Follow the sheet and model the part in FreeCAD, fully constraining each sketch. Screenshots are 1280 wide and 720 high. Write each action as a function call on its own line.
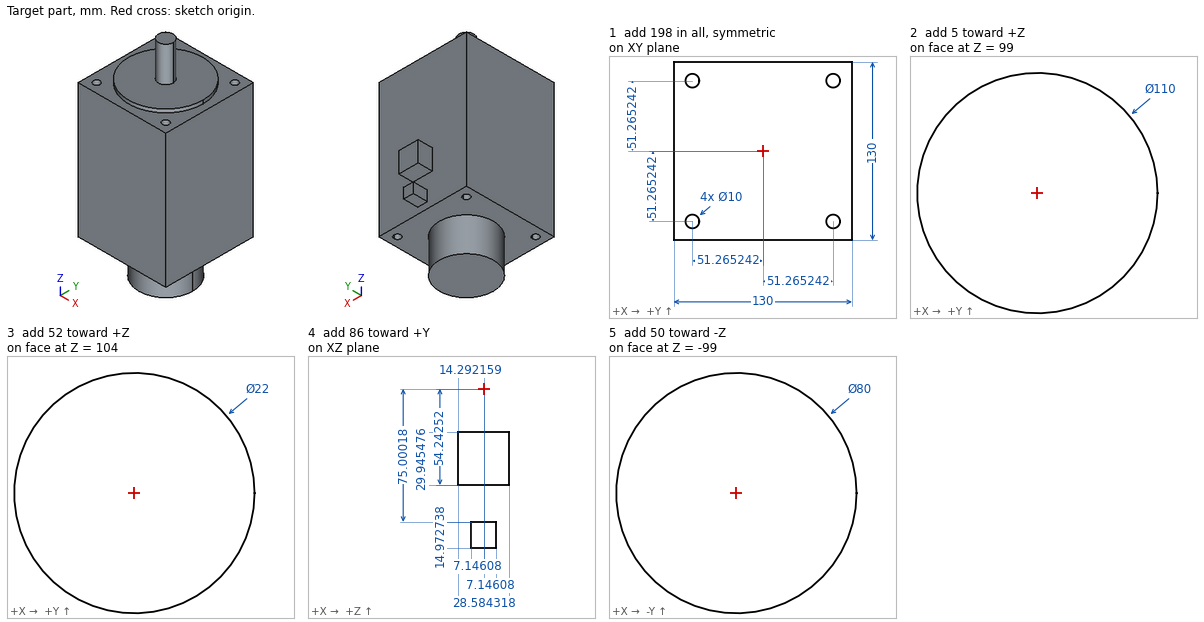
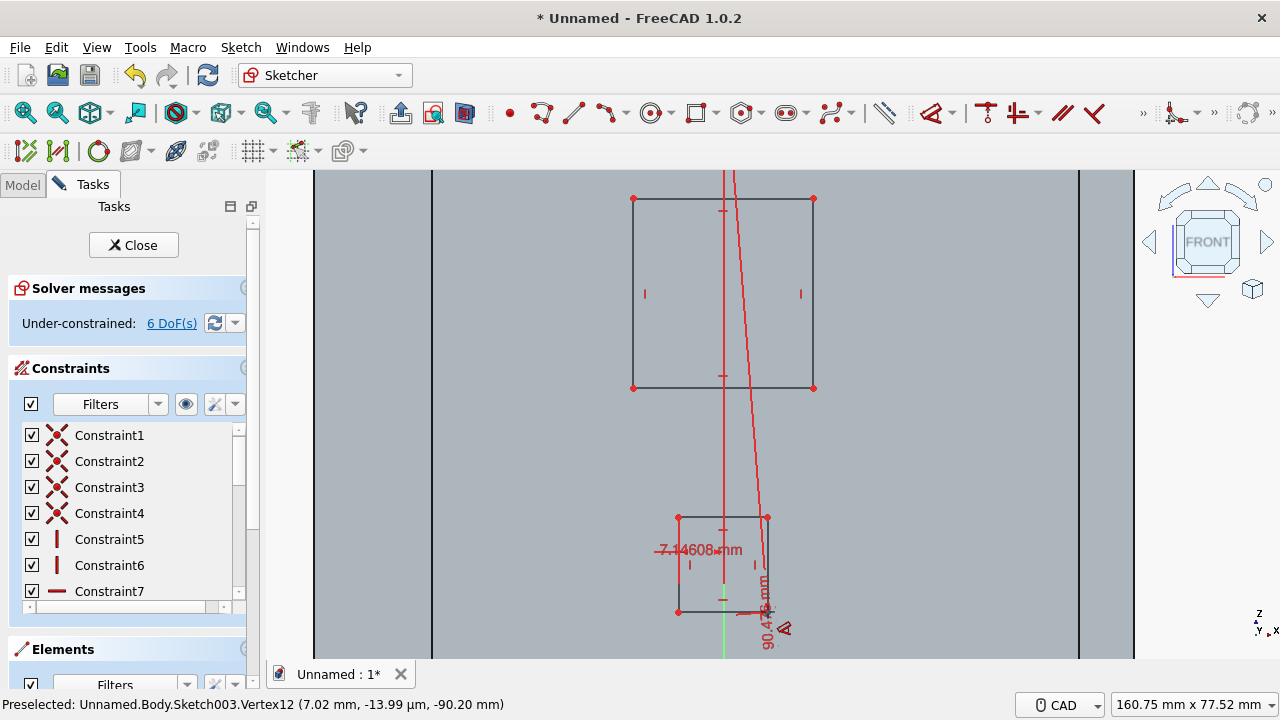
key(Escape)
key(Escape)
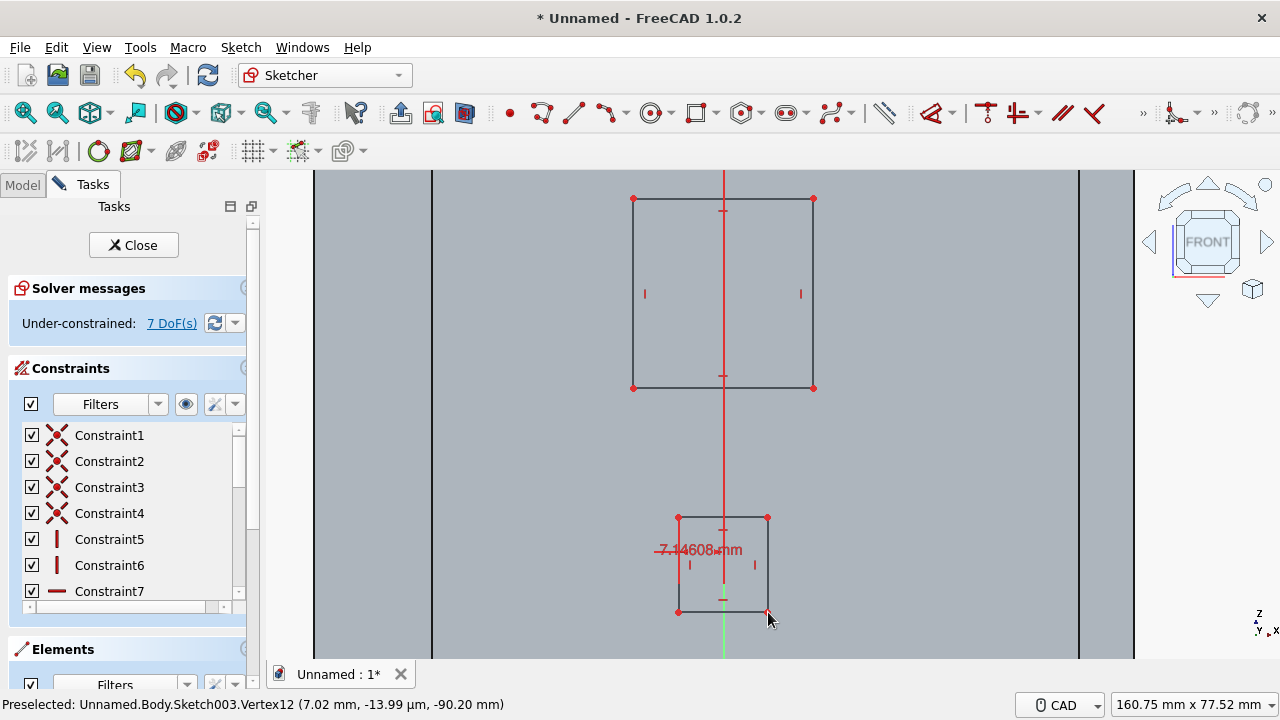
click(768, 612)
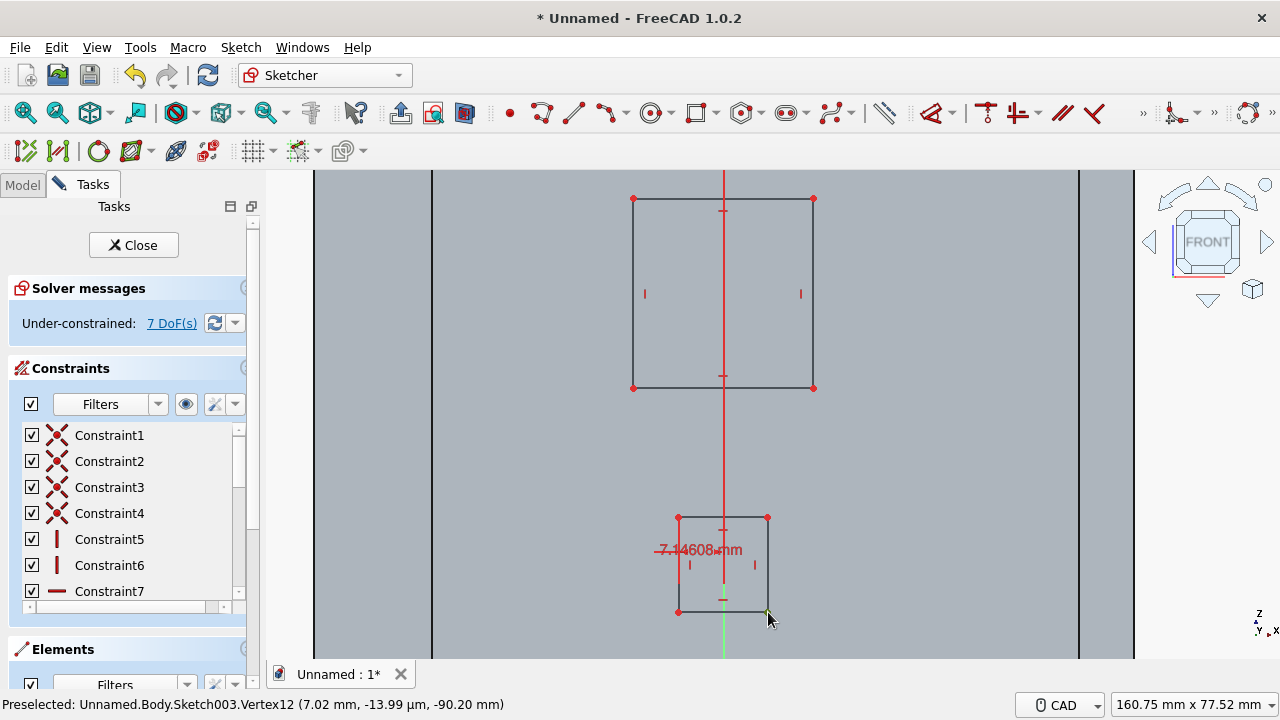
click(954, 114)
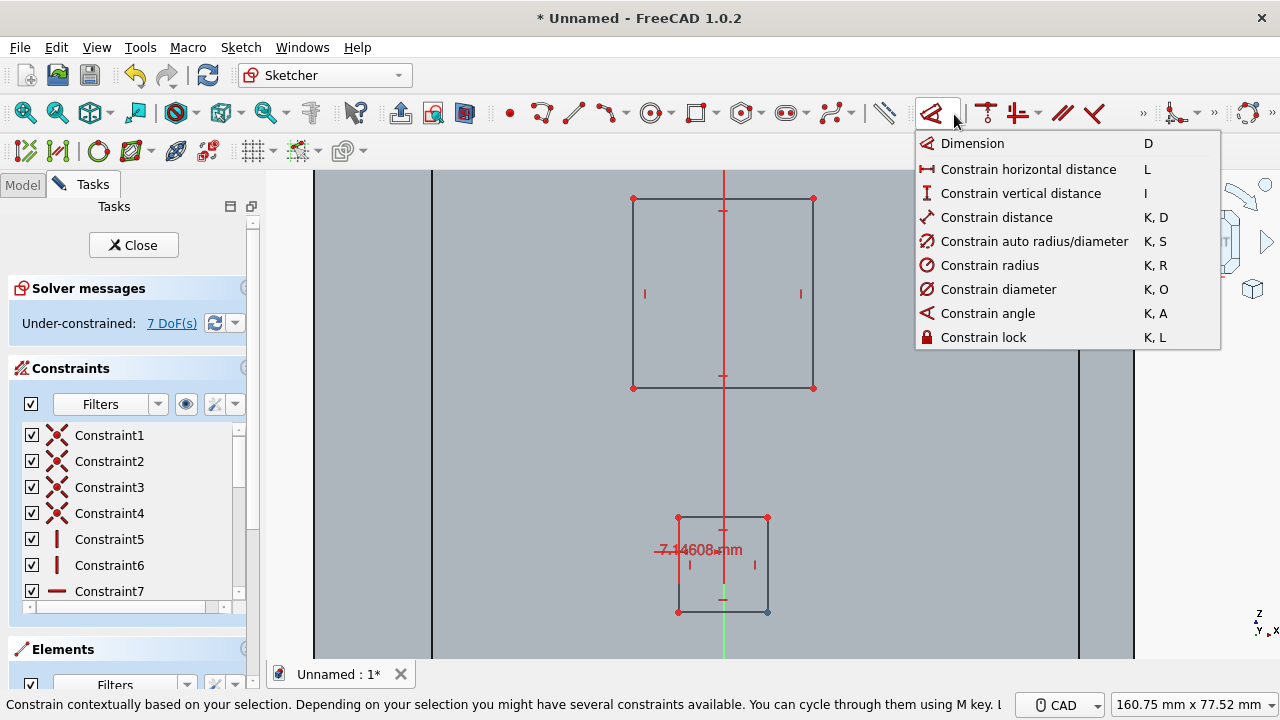
click(1068, 169)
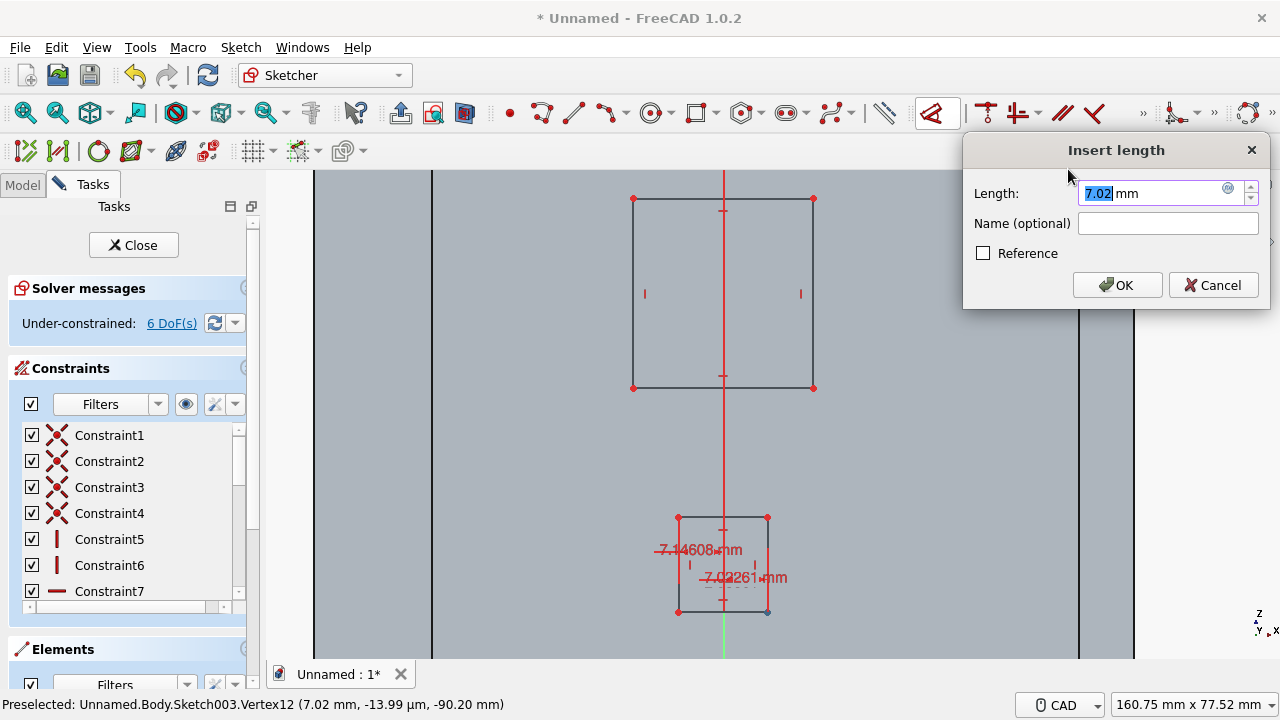
text(7.14608)
key(Return)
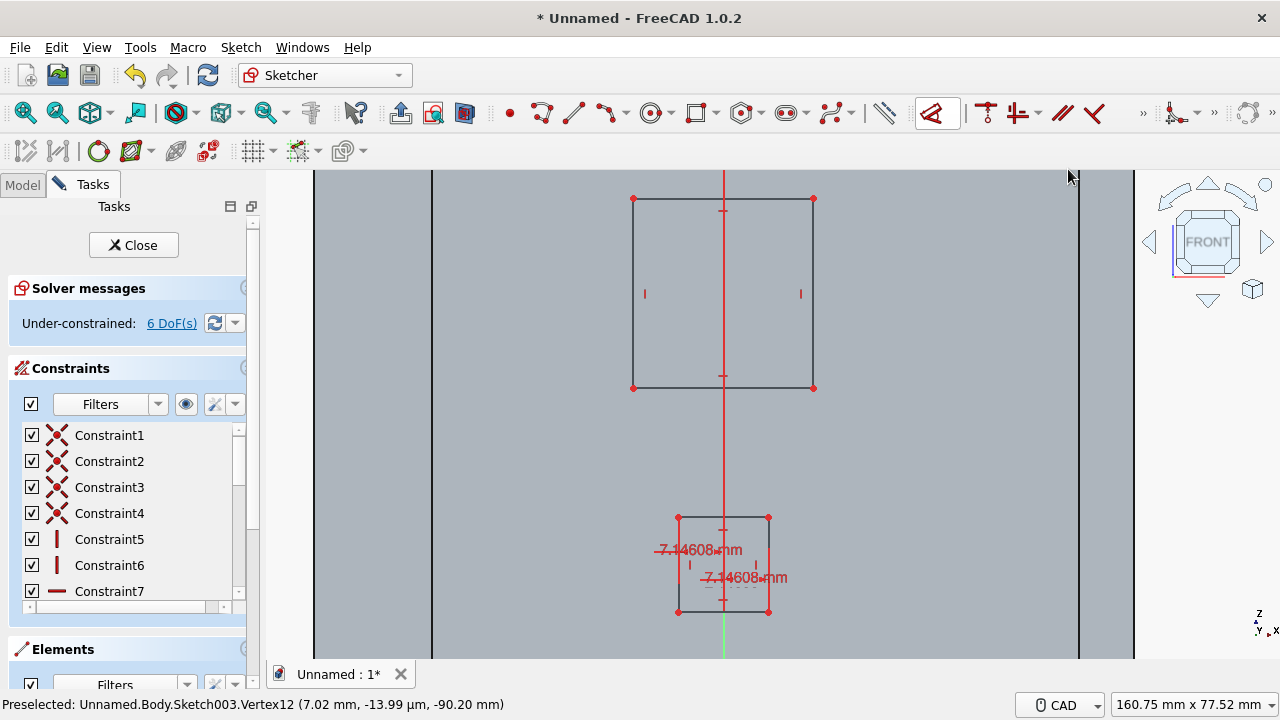
click(633, 255)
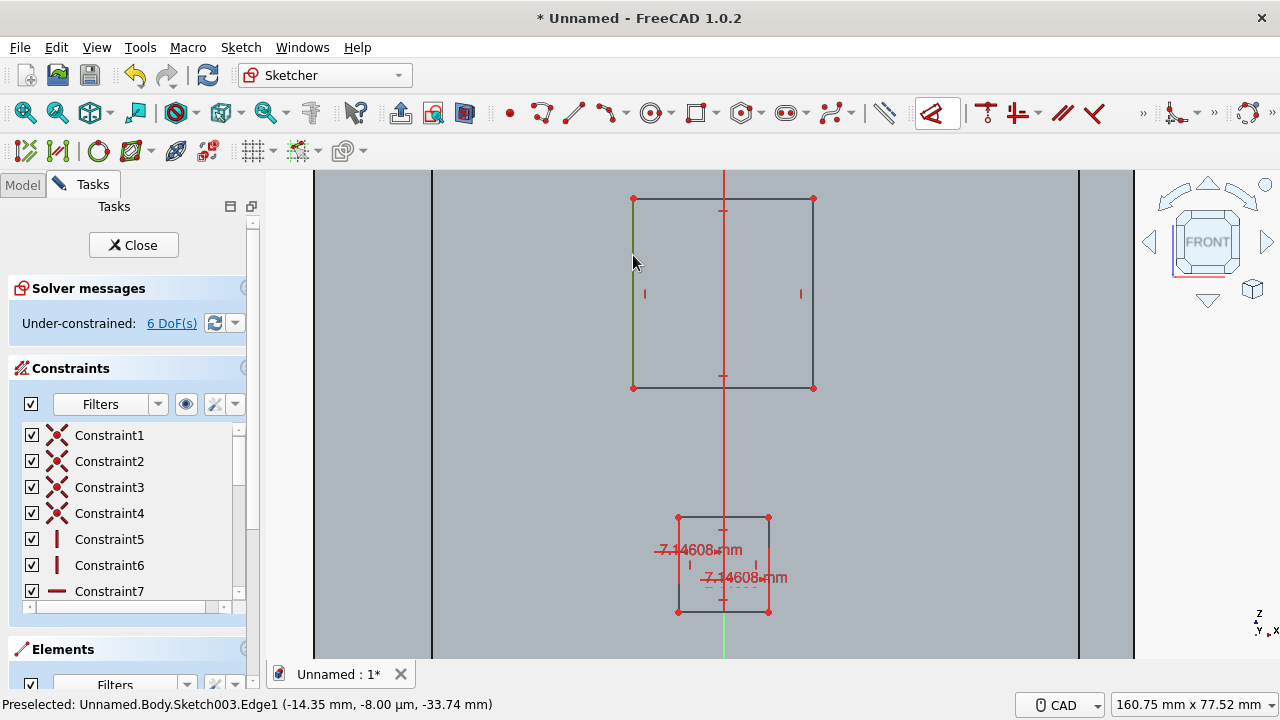
key(i)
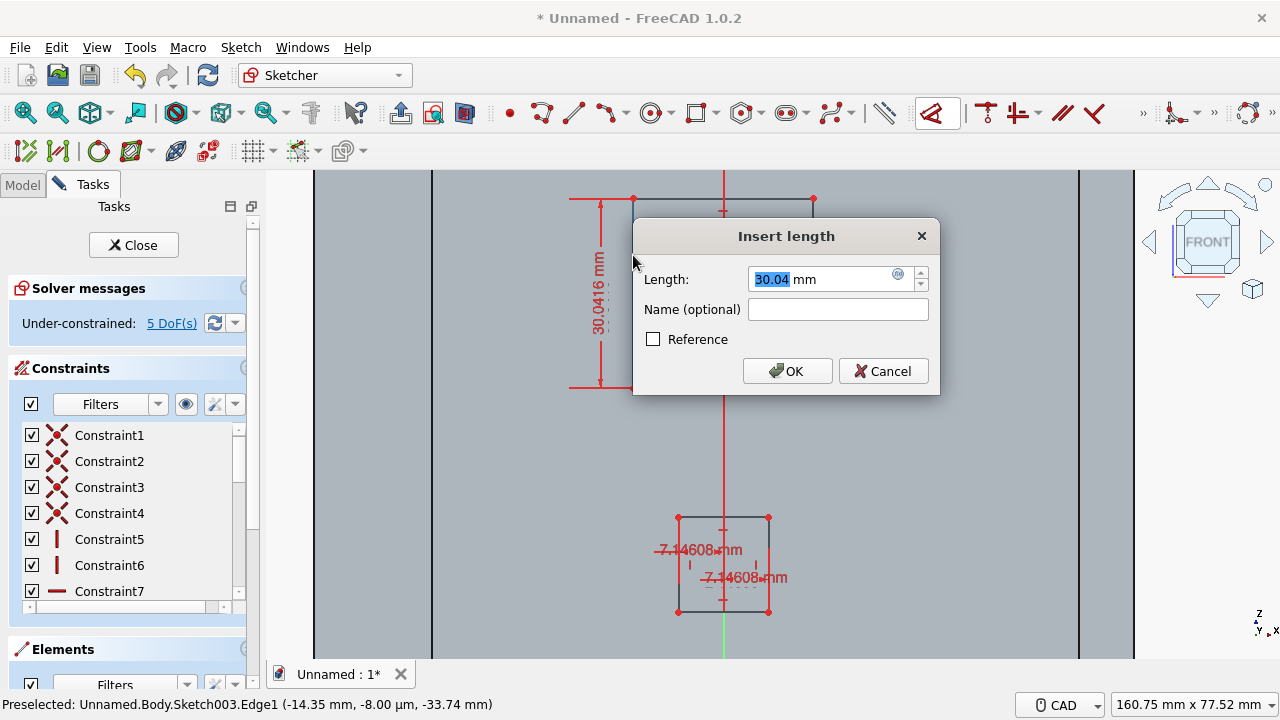
text(29.945476)
key(Return)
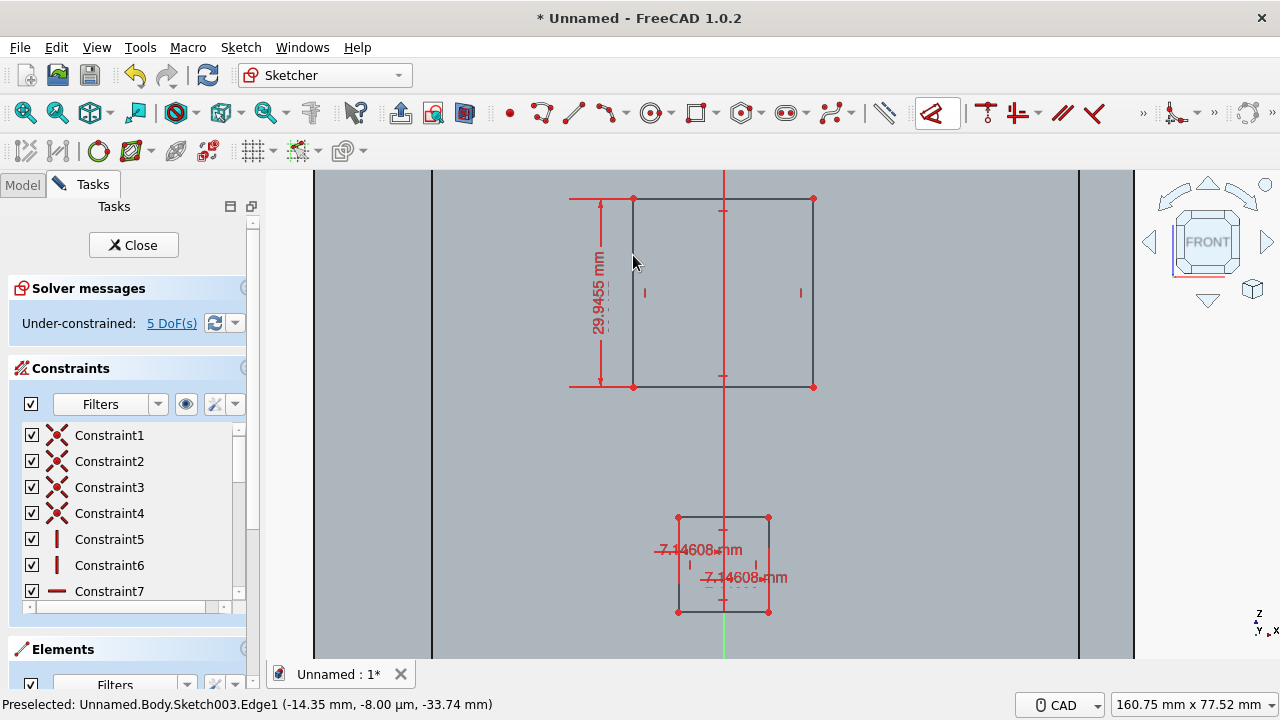
click(687, 387)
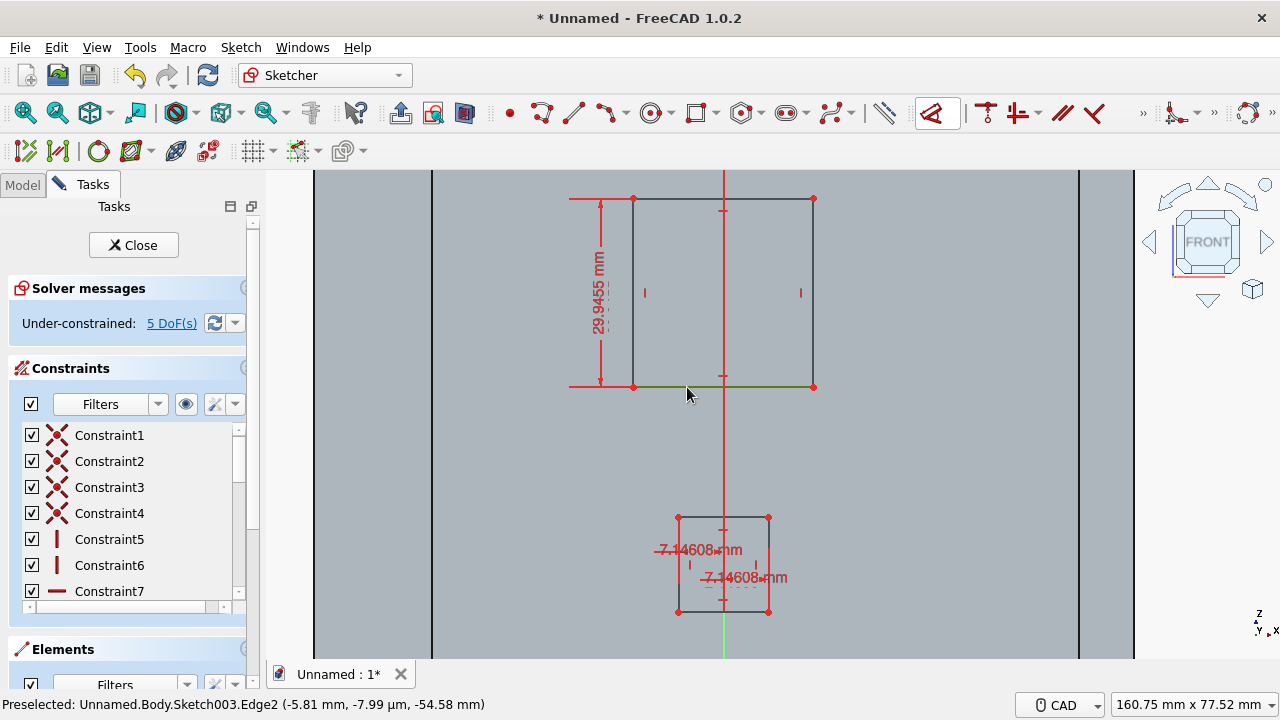
key(l)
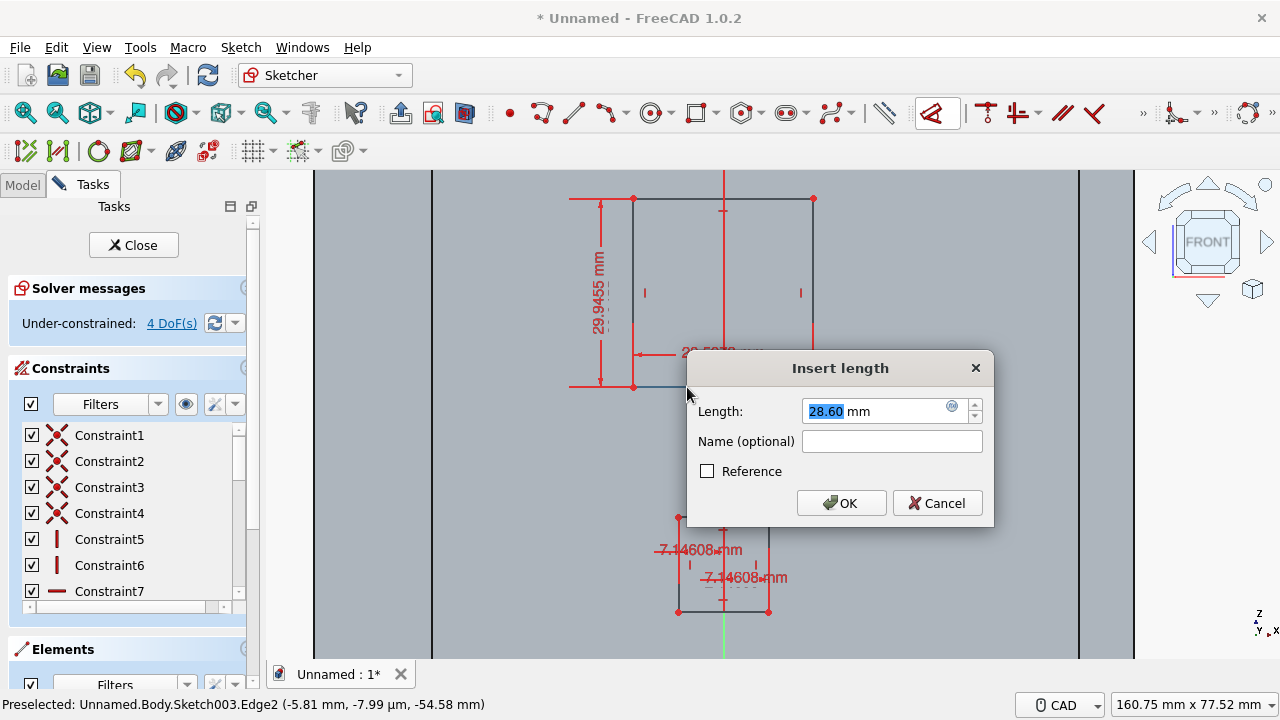
text(28.584318)
key(Return)